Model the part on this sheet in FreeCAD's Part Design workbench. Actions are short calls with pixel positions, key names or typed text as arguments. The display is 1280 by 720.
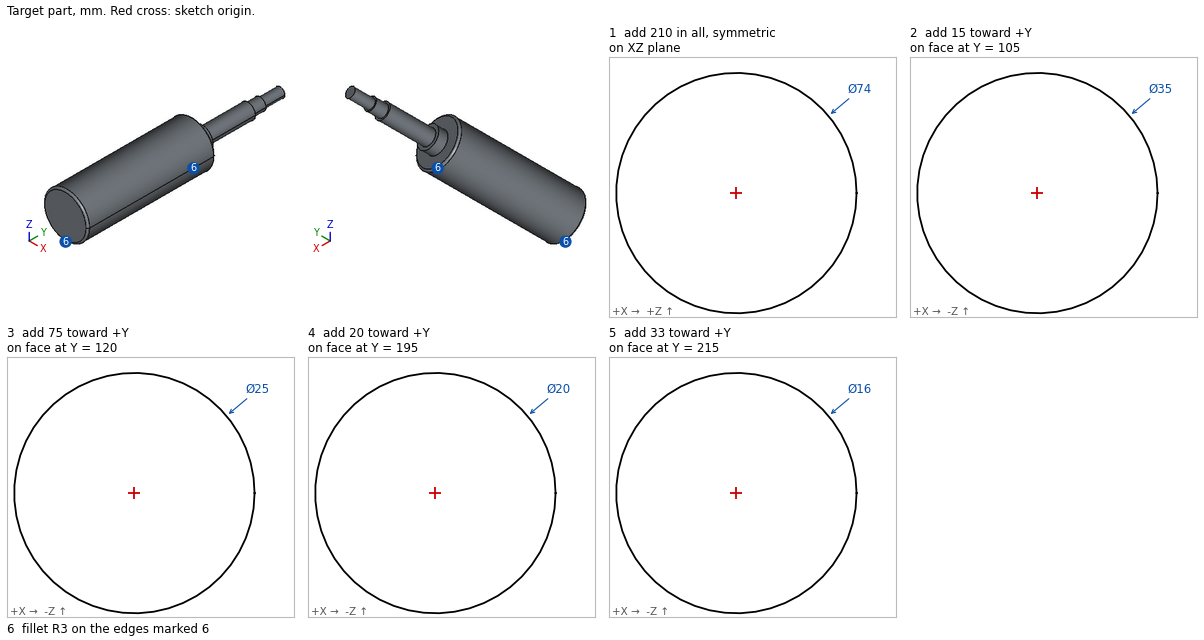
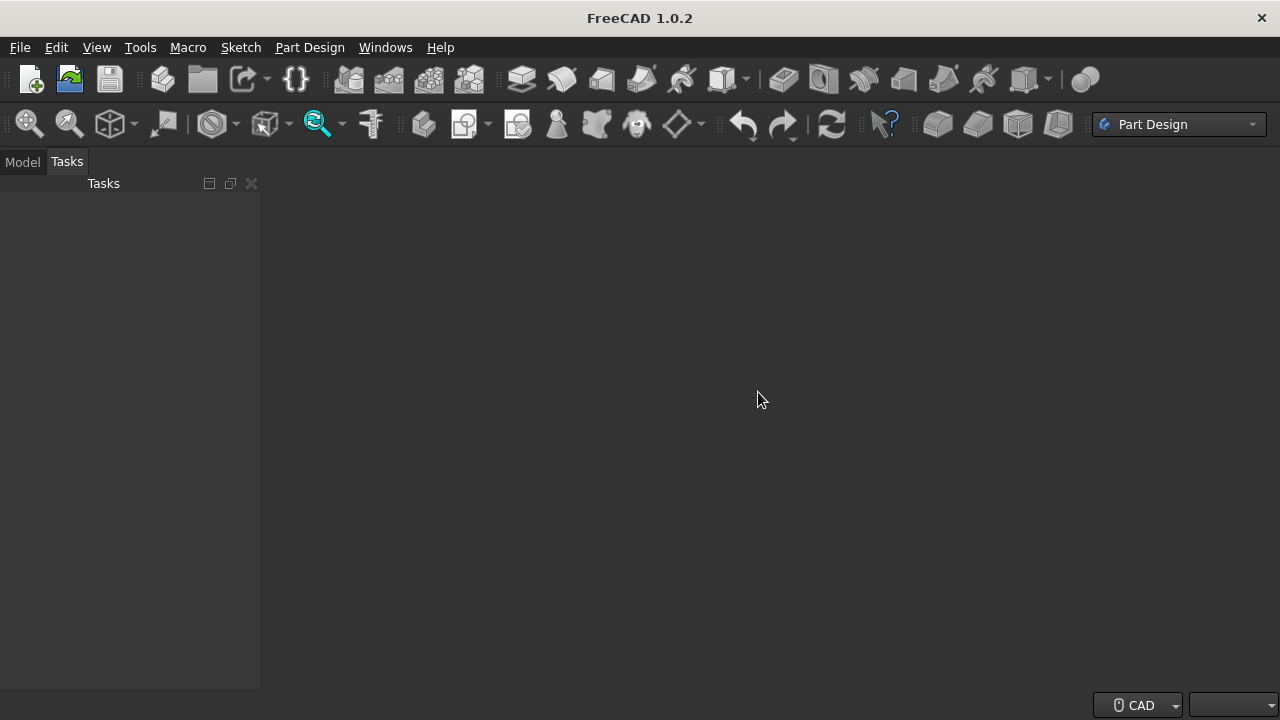
click(30, 80)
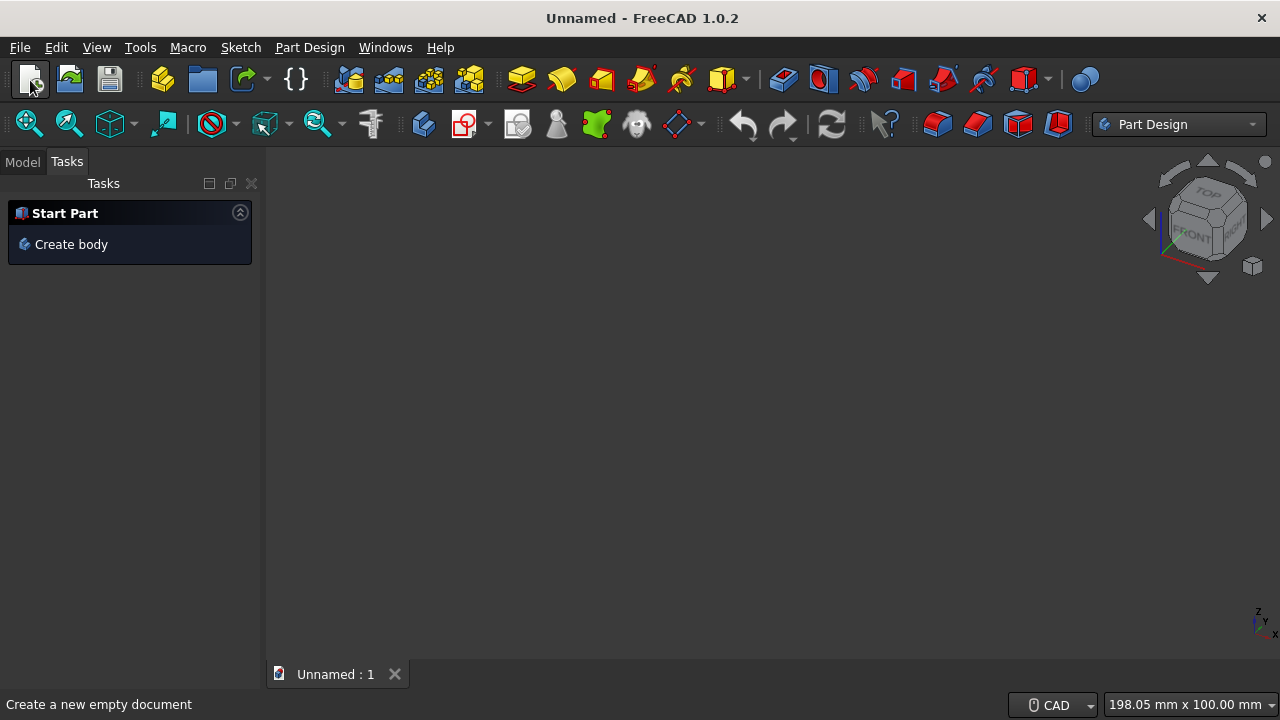
click(464, 124)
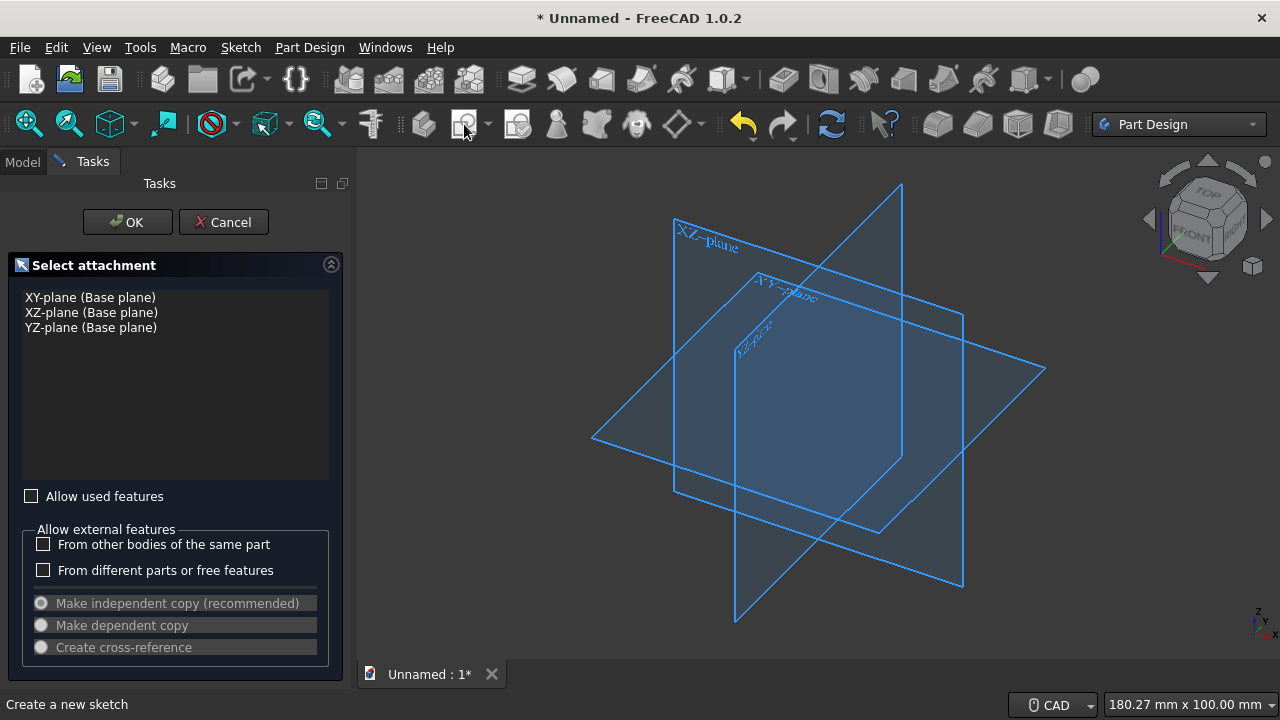
click(82, 312)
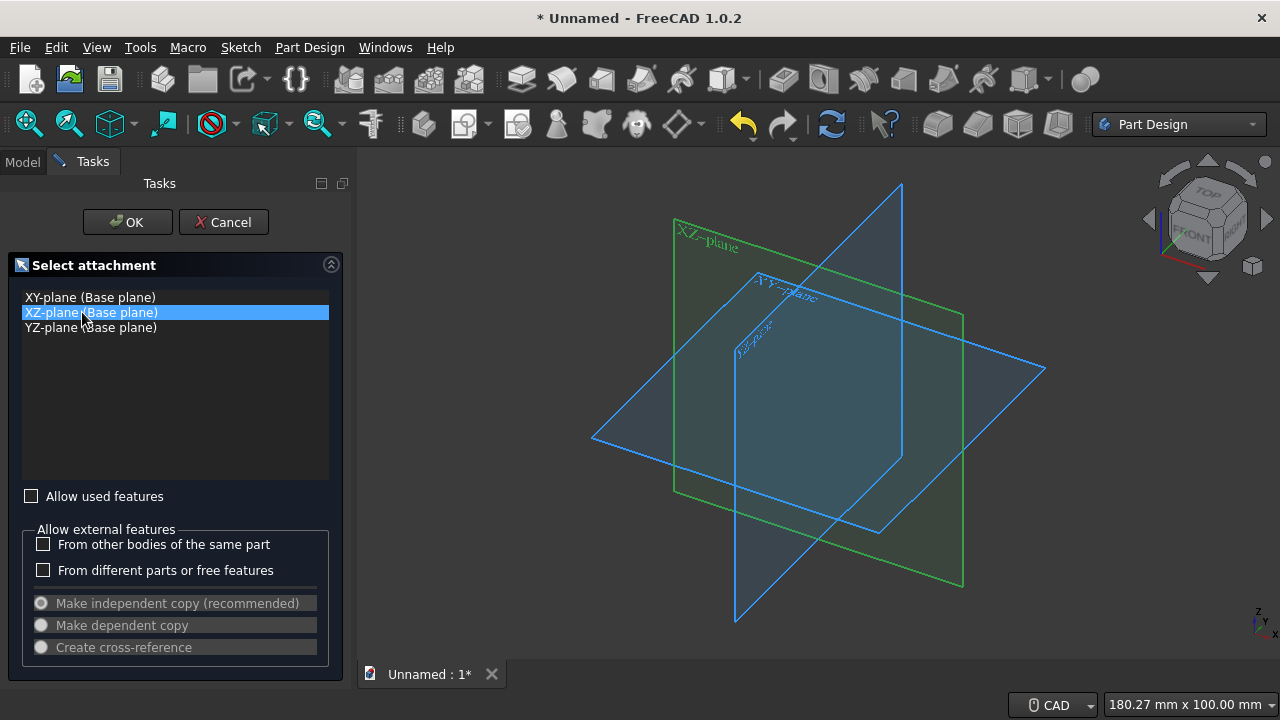
click(128, 222)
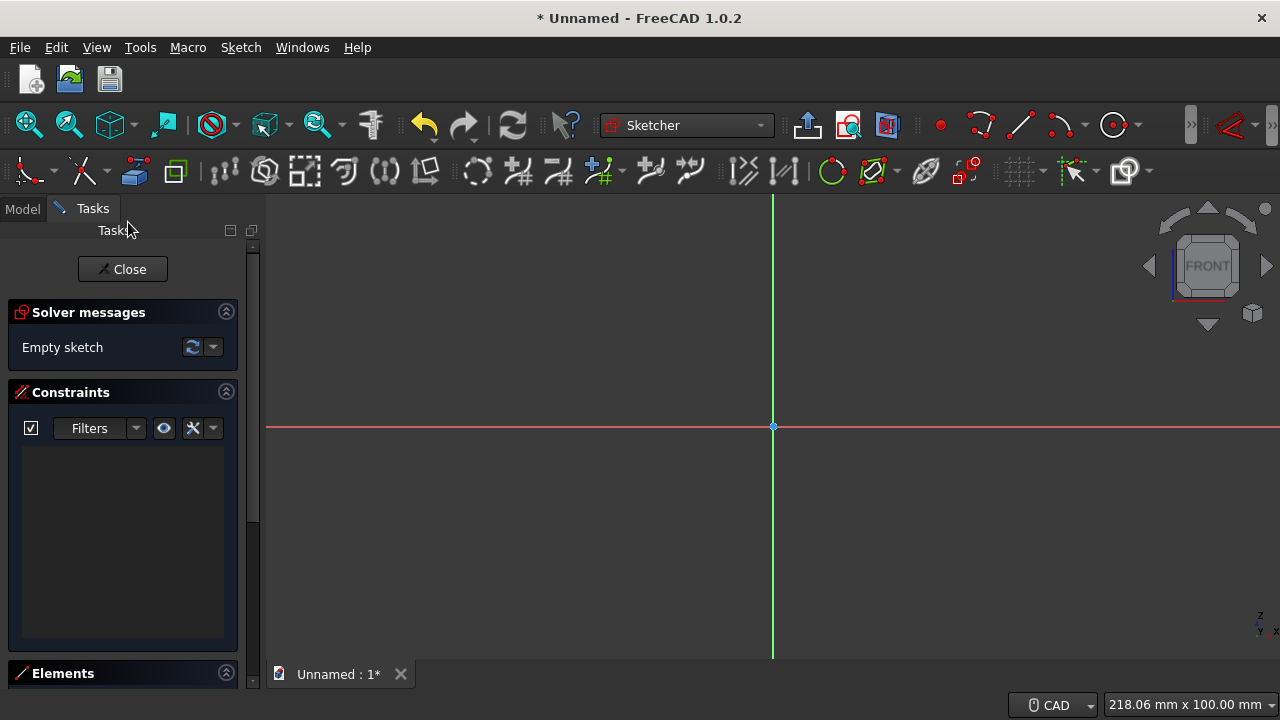
key(g)
key(c)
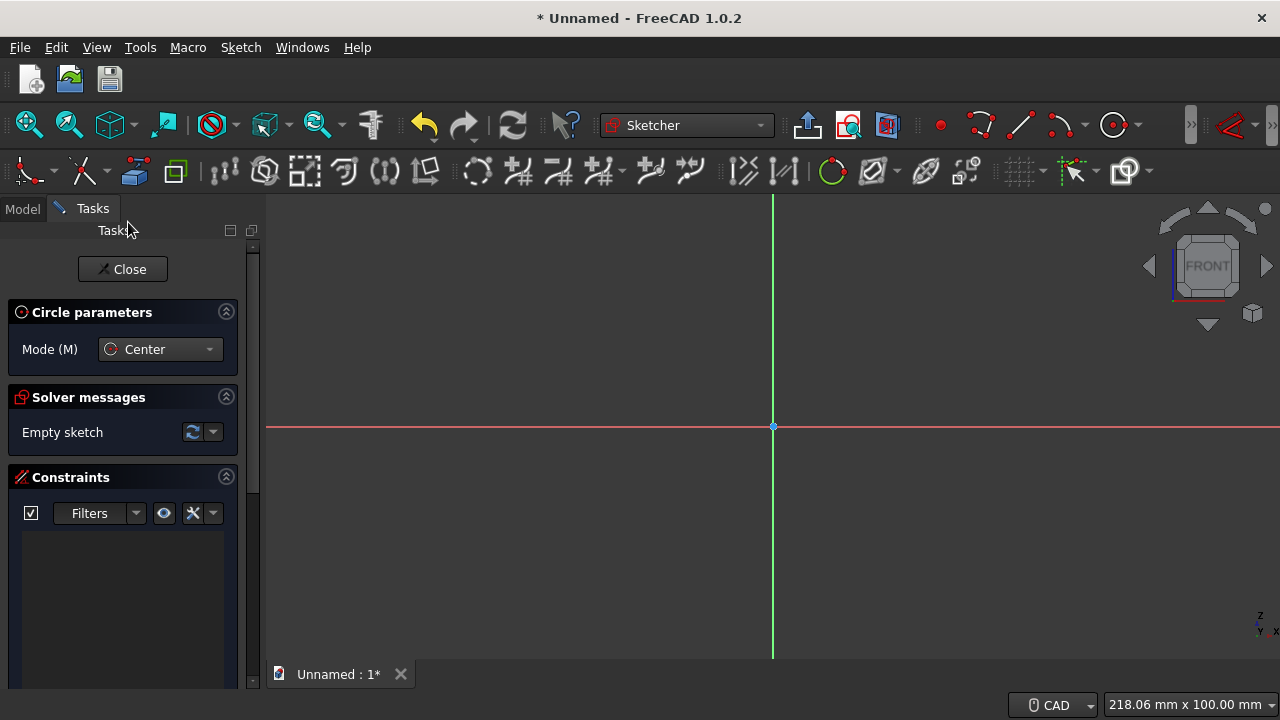
click(773, 426)
move(895, 305)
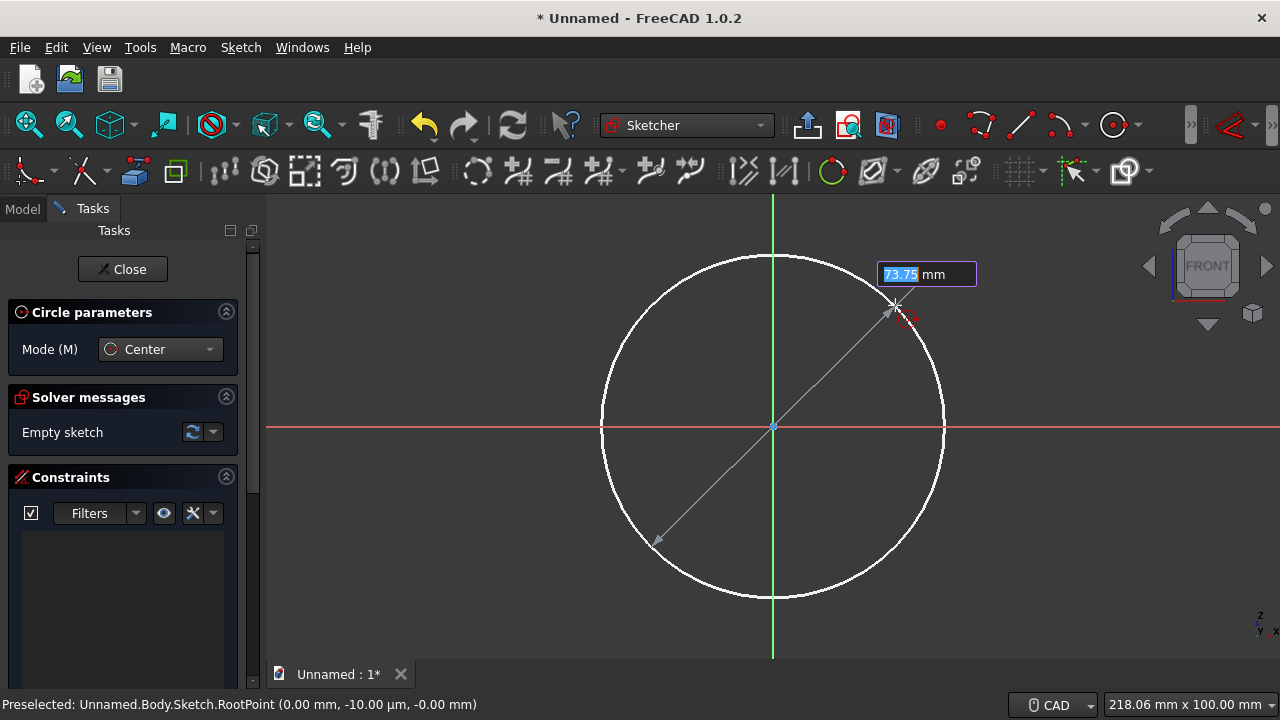
text(74)
key(Return)
key(Escape)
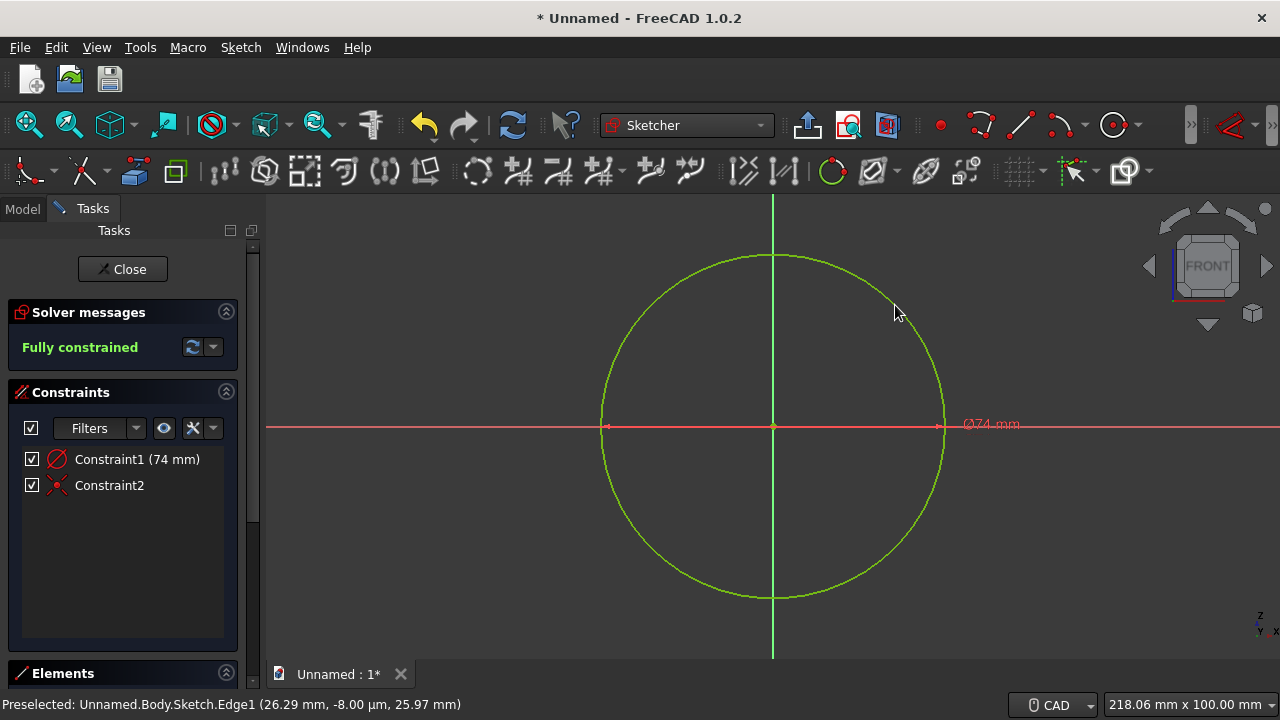
click(123, 269)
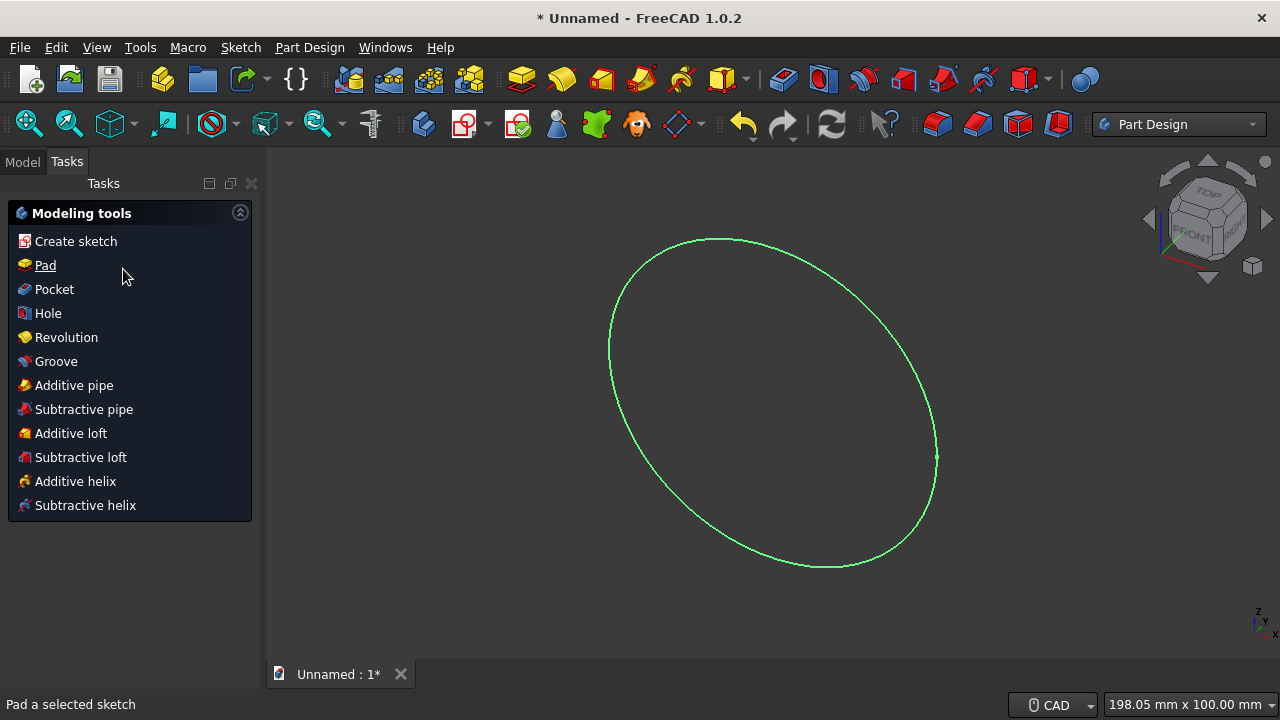
click(522, 80)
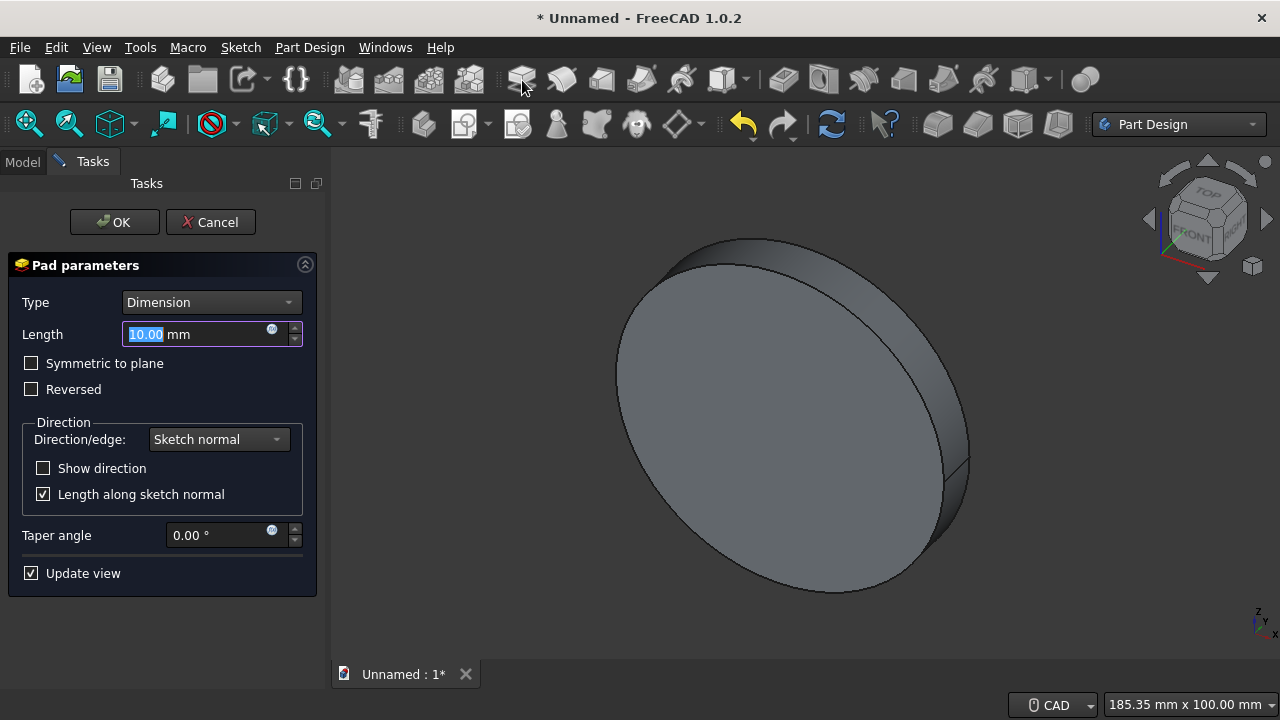
text(210)
key(Tab)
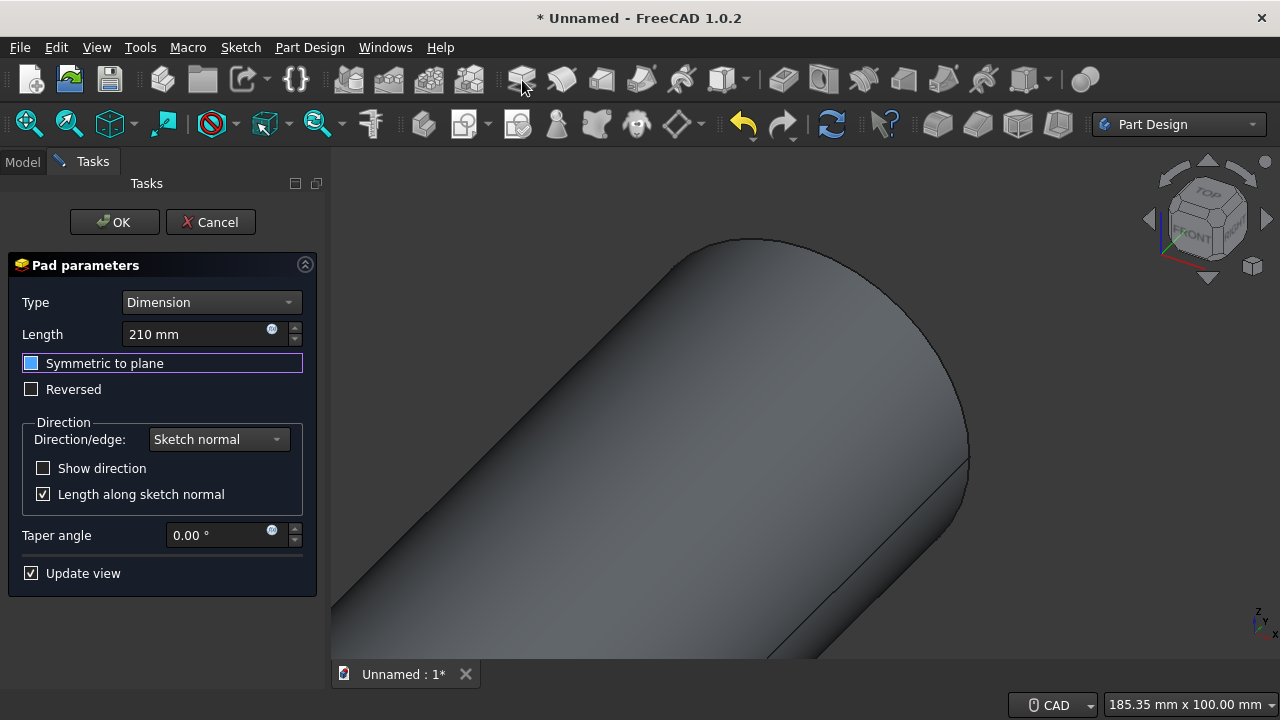
click(30, 363)